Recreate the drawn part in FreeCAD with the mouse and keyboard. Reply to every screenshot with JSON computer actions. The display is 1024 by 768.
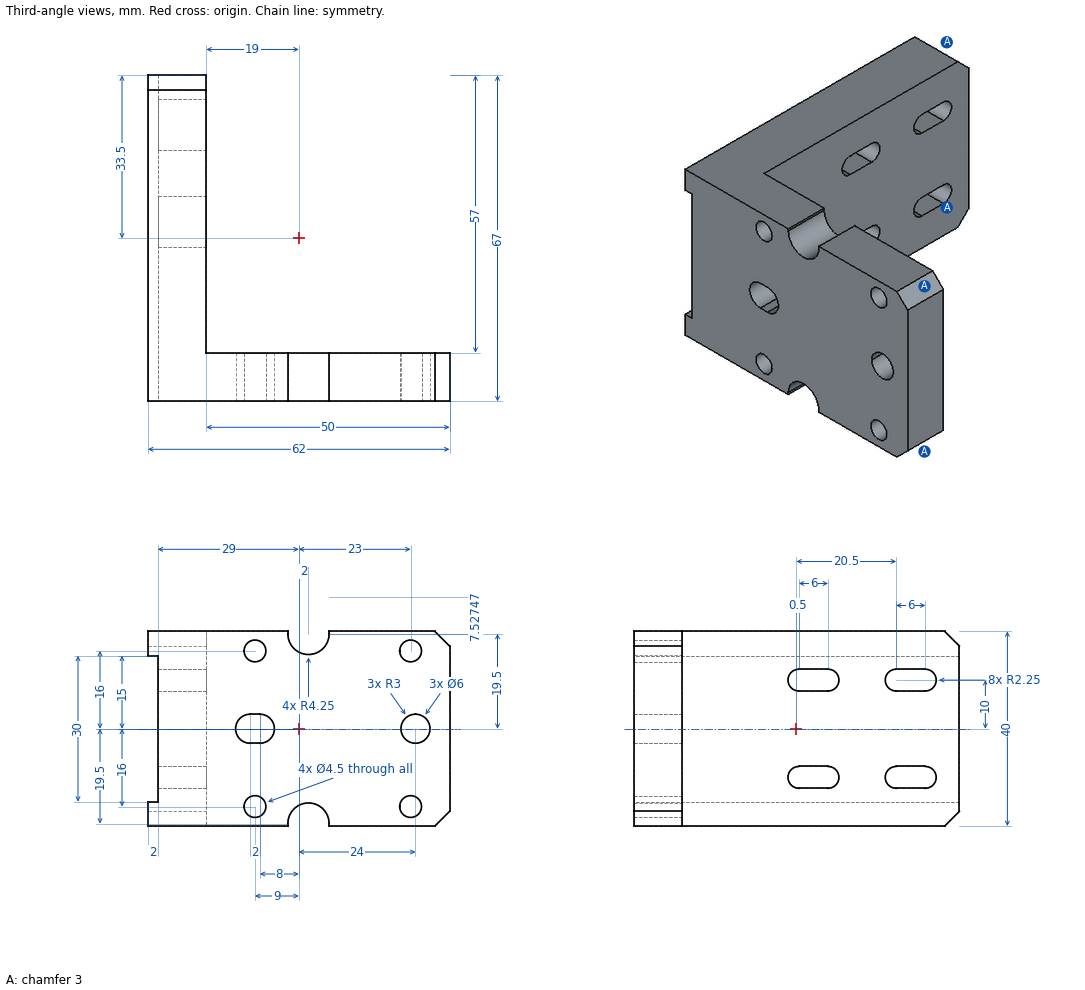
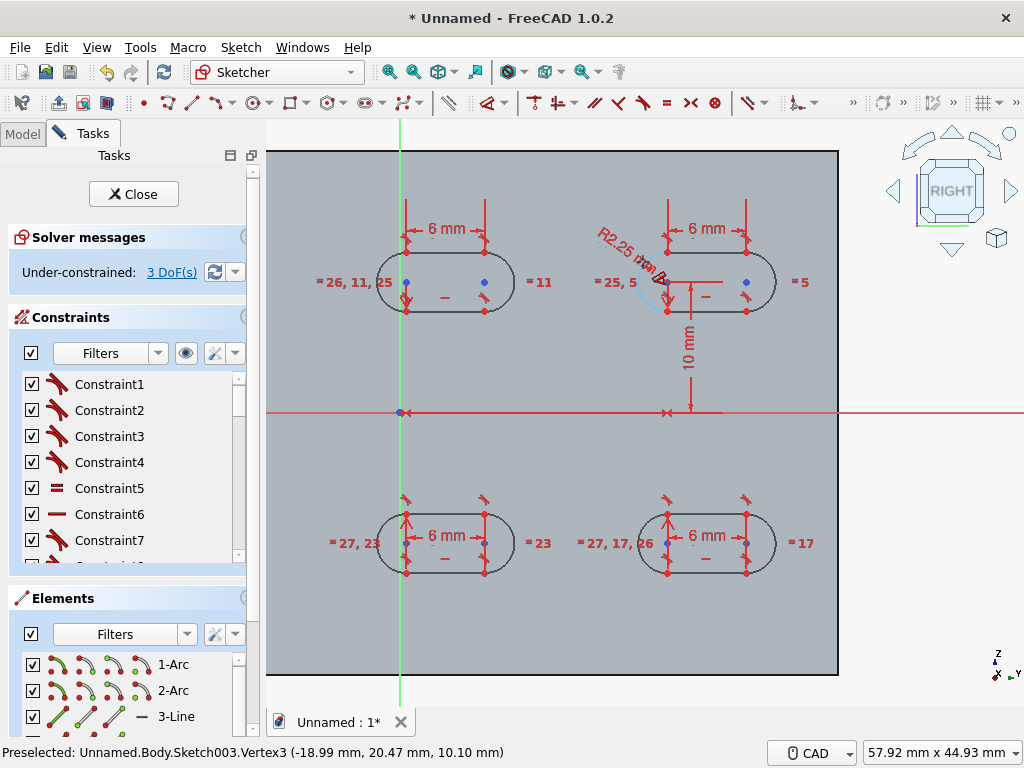
{"action": "left_click", "coordinate": [406, 282]}
{"action": "left_click", "coordinate": [366, 348]}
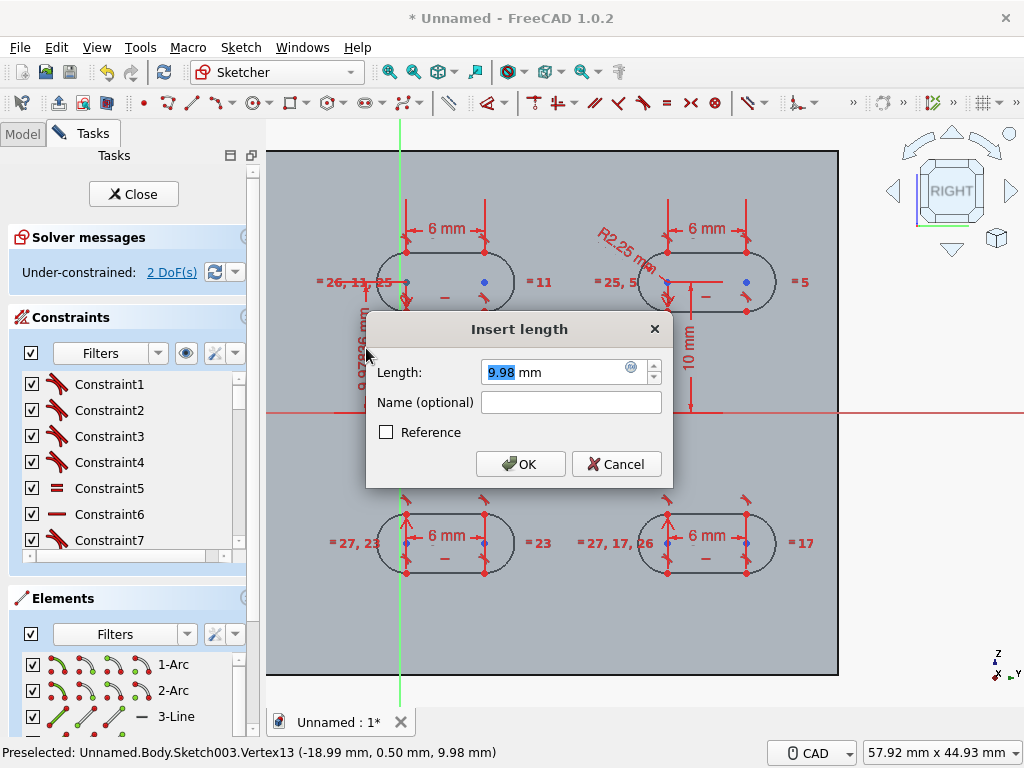
{"action": "type", "text": "10"}
{"action": "key", "text": "Return"}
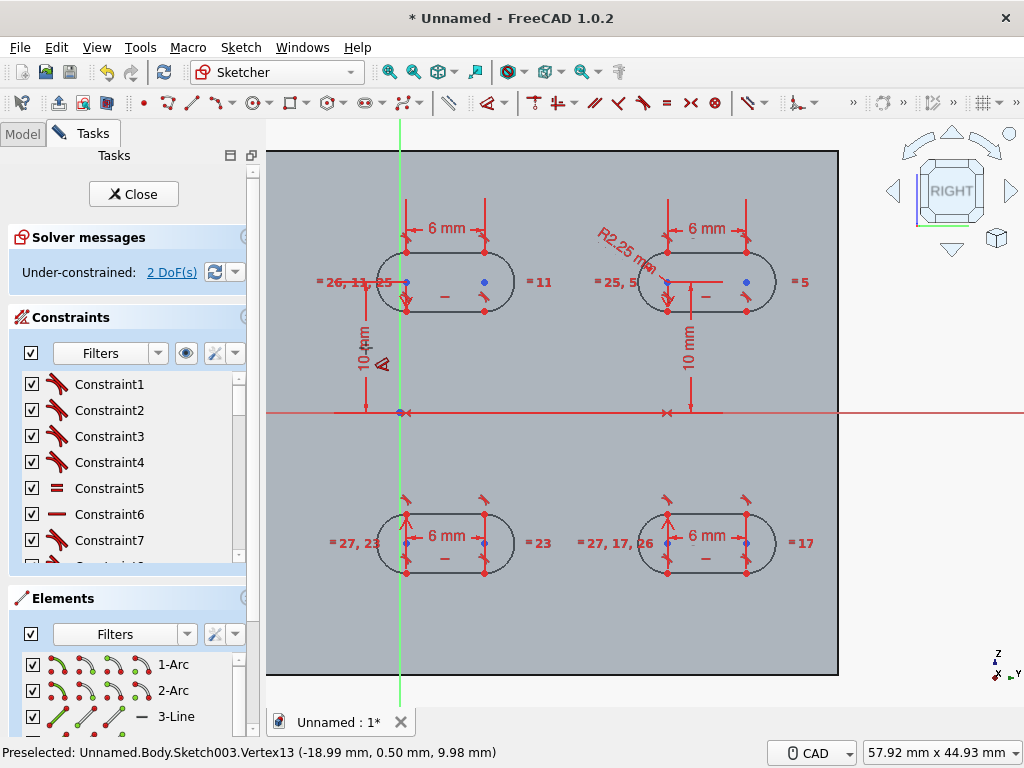
{"action": "scroll", "coordinate": [406, 253], "scroll_direction": "up", "scroll_amount": 10}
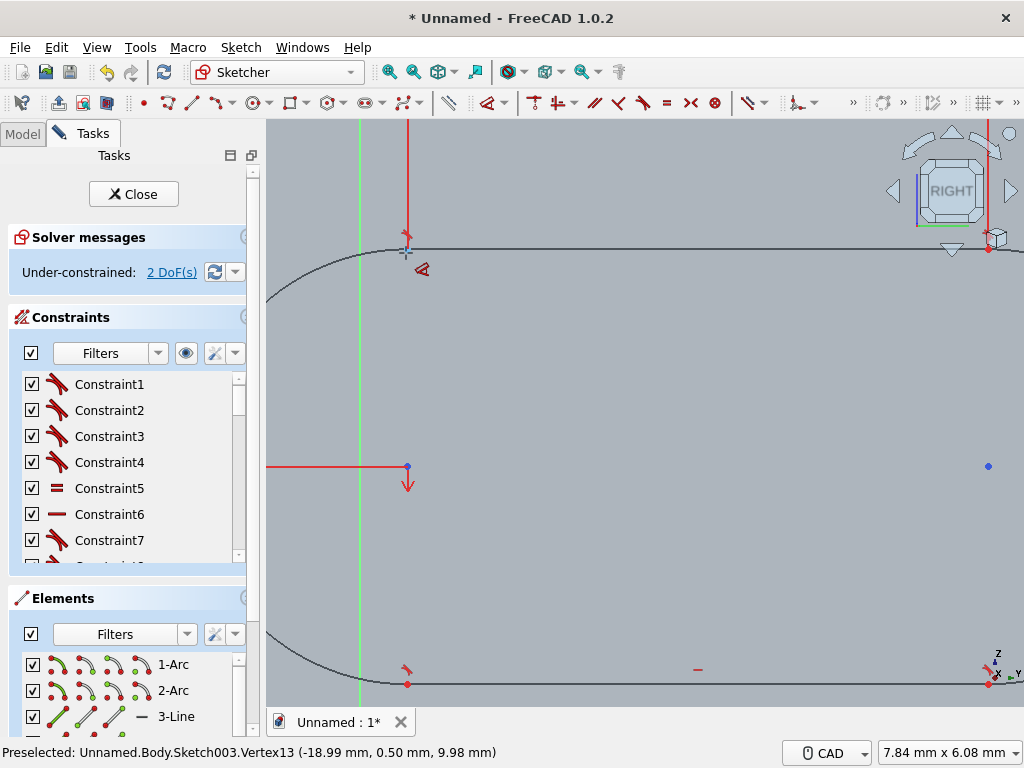
{"action": "left_click", "coordinate": [408, 249]}
{"action": "left_click", "coordinate": [384, 215]}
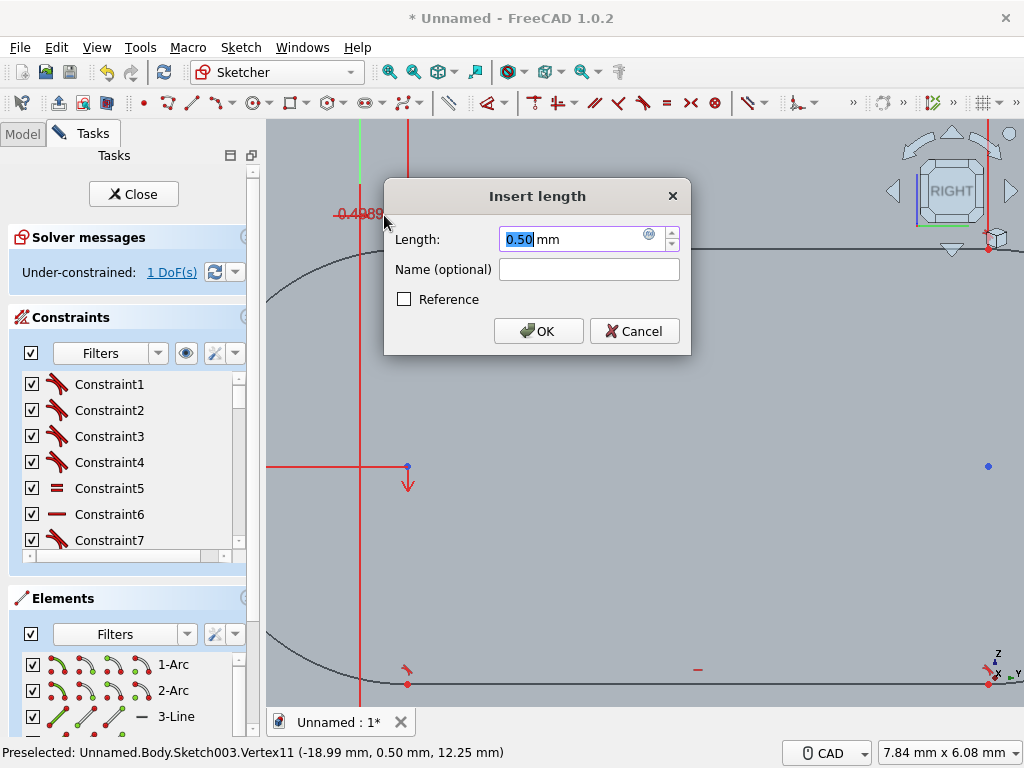
{"action": "type", "text": "0.5"}
{"action": "key", "text": "Return"}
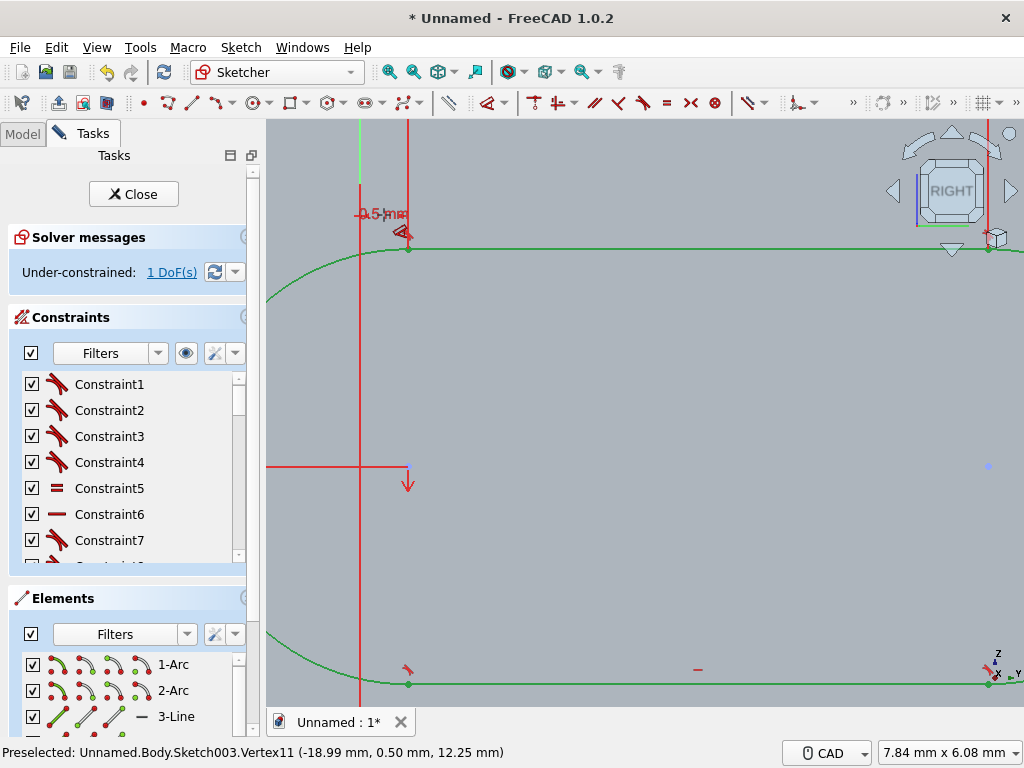
{"action": "scroll", "coordinate": [406, 253], "scroll_direction": "down", "scroll_amount": 10}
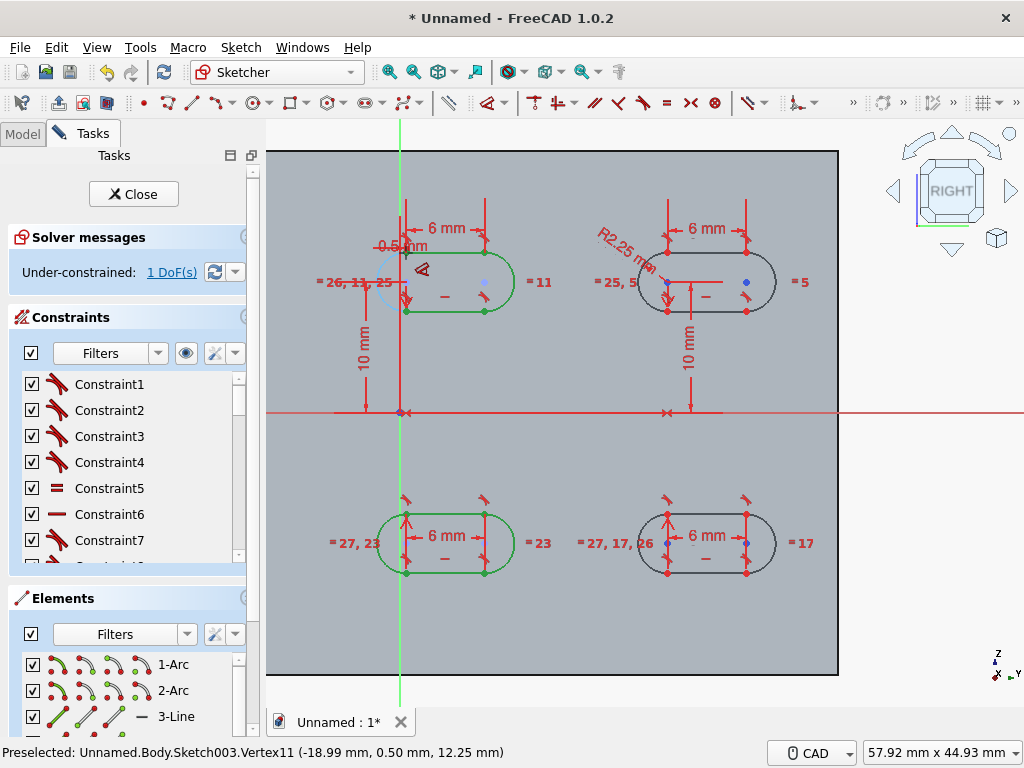
{"action": "left_click", "coordinate": [668, 253]}
{"action": "left_click", "coordinate": [534, 219]}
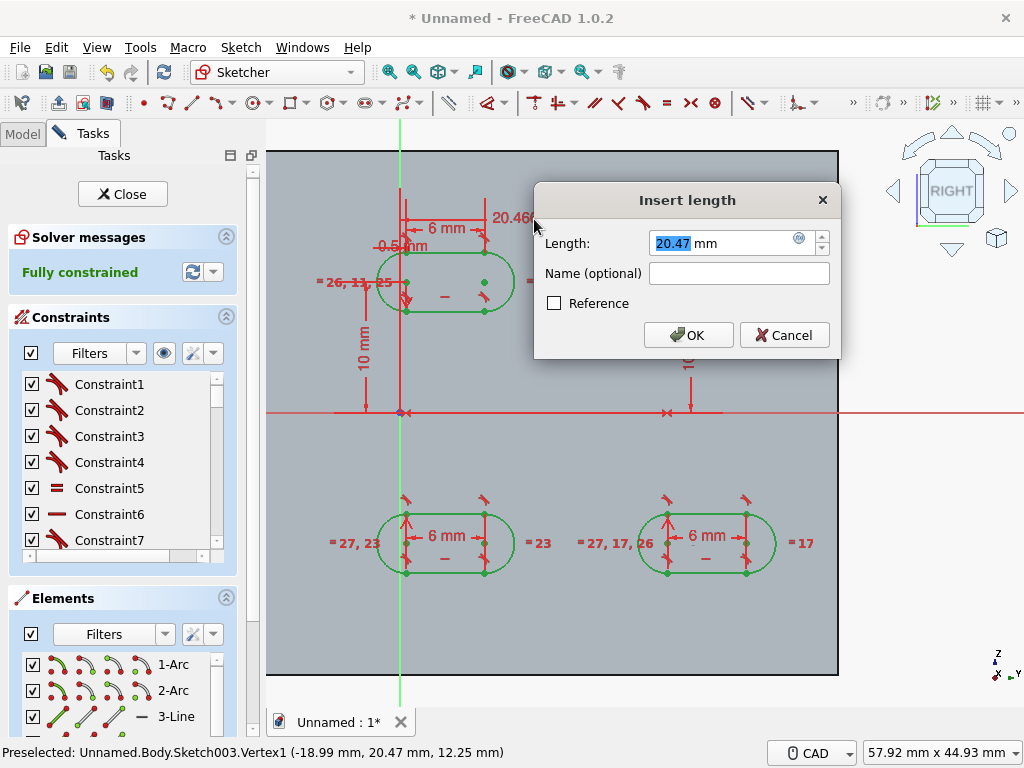
{"action": "type", "text": "20.5"}
{"action": "key", "text": "Return"}
{"action": "key", "text": "Escape"}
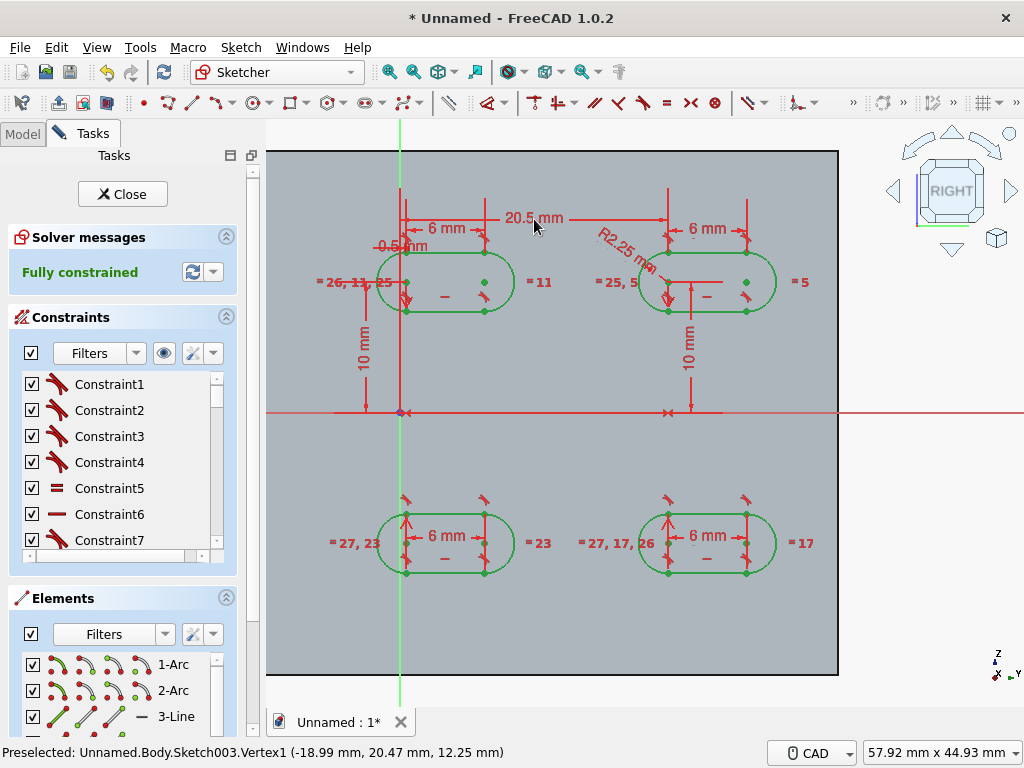
{"action": "left_click", "coordinate": [123, 194]}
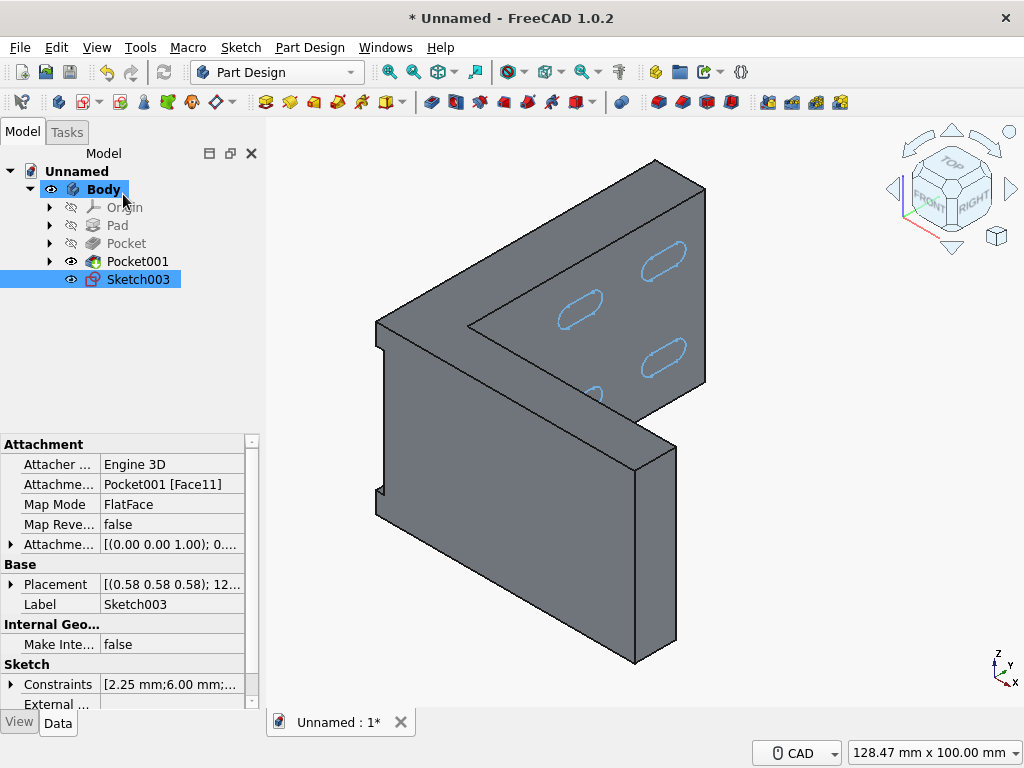
{"action": "left_click", "coordinate": [432, 102]}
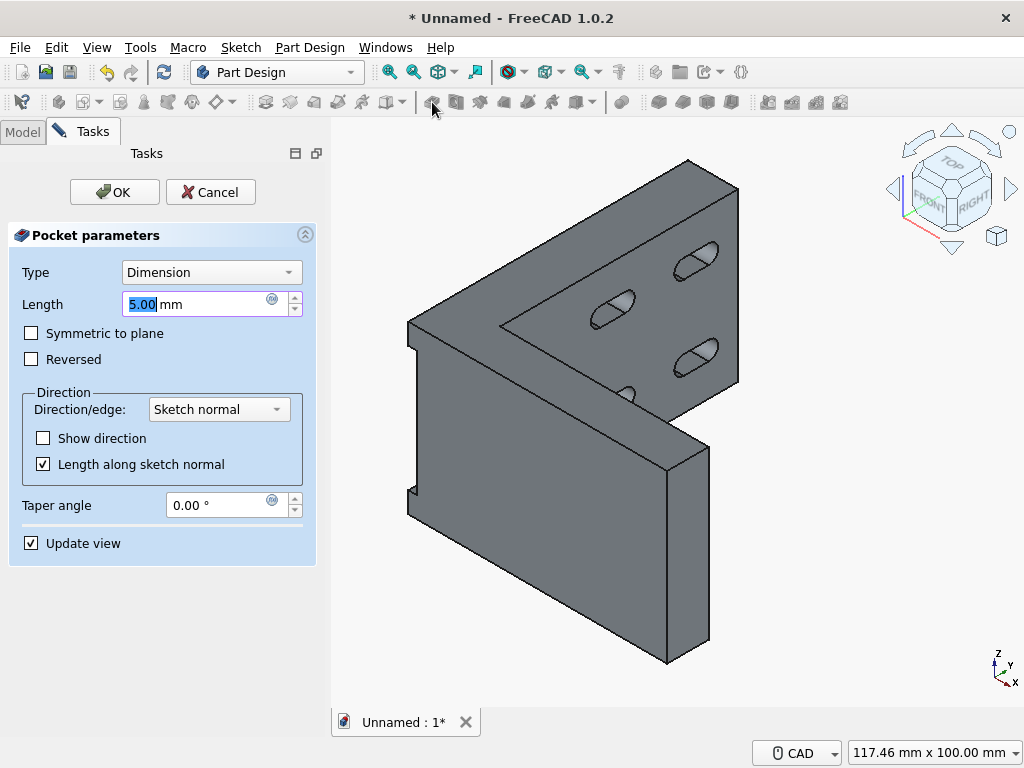
{"action": "left_click", "coordinate": [212, 272]}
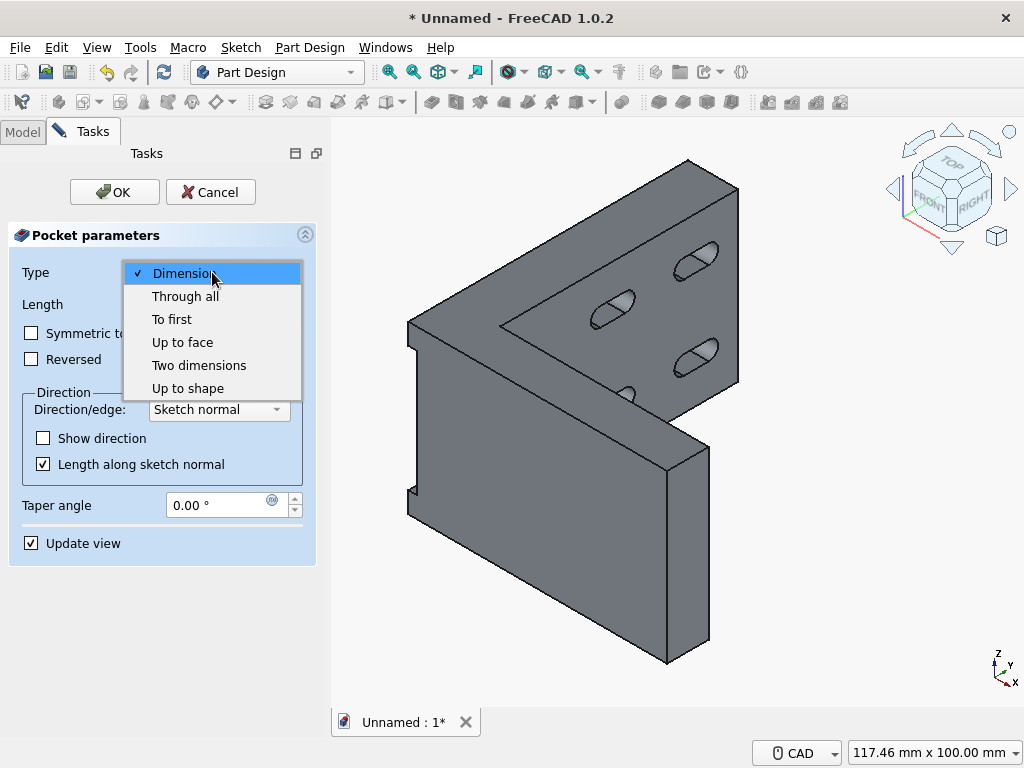
{"action": "left_click", "coordinate": [212, 296]}